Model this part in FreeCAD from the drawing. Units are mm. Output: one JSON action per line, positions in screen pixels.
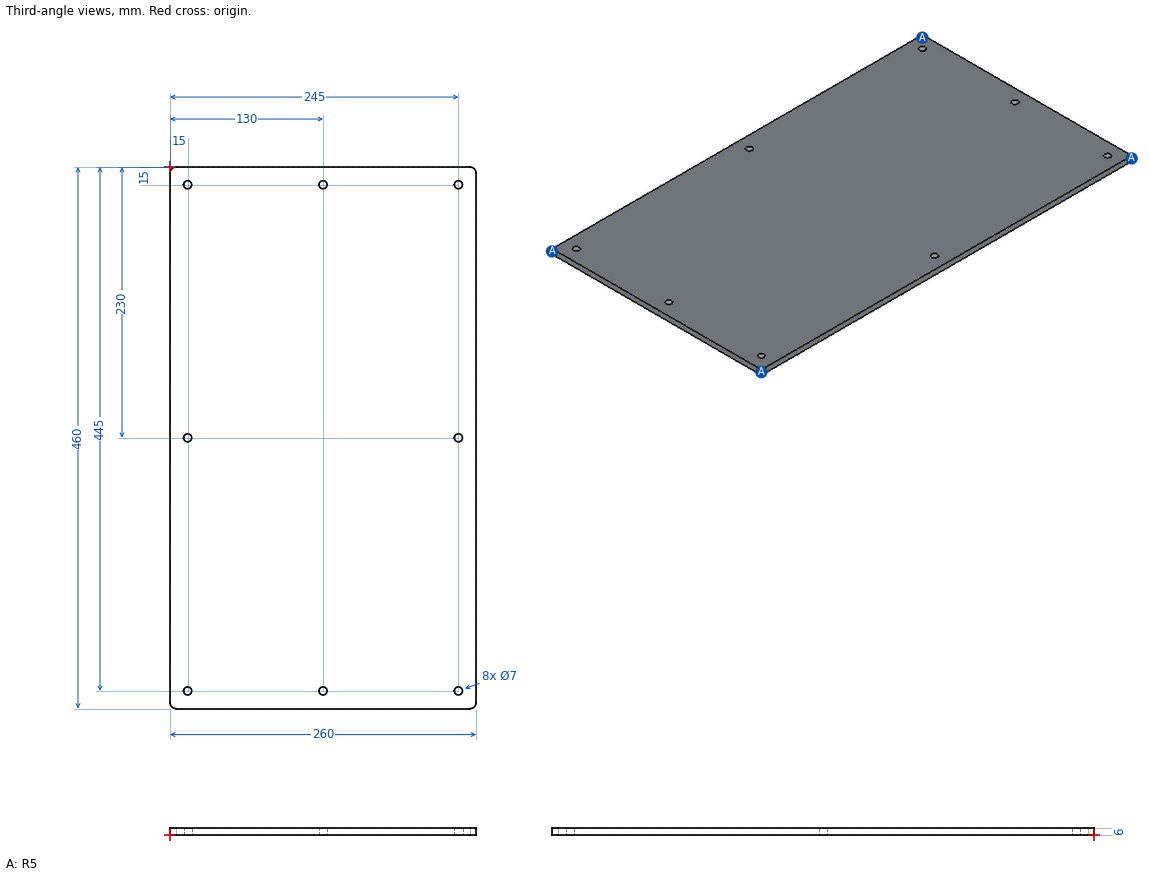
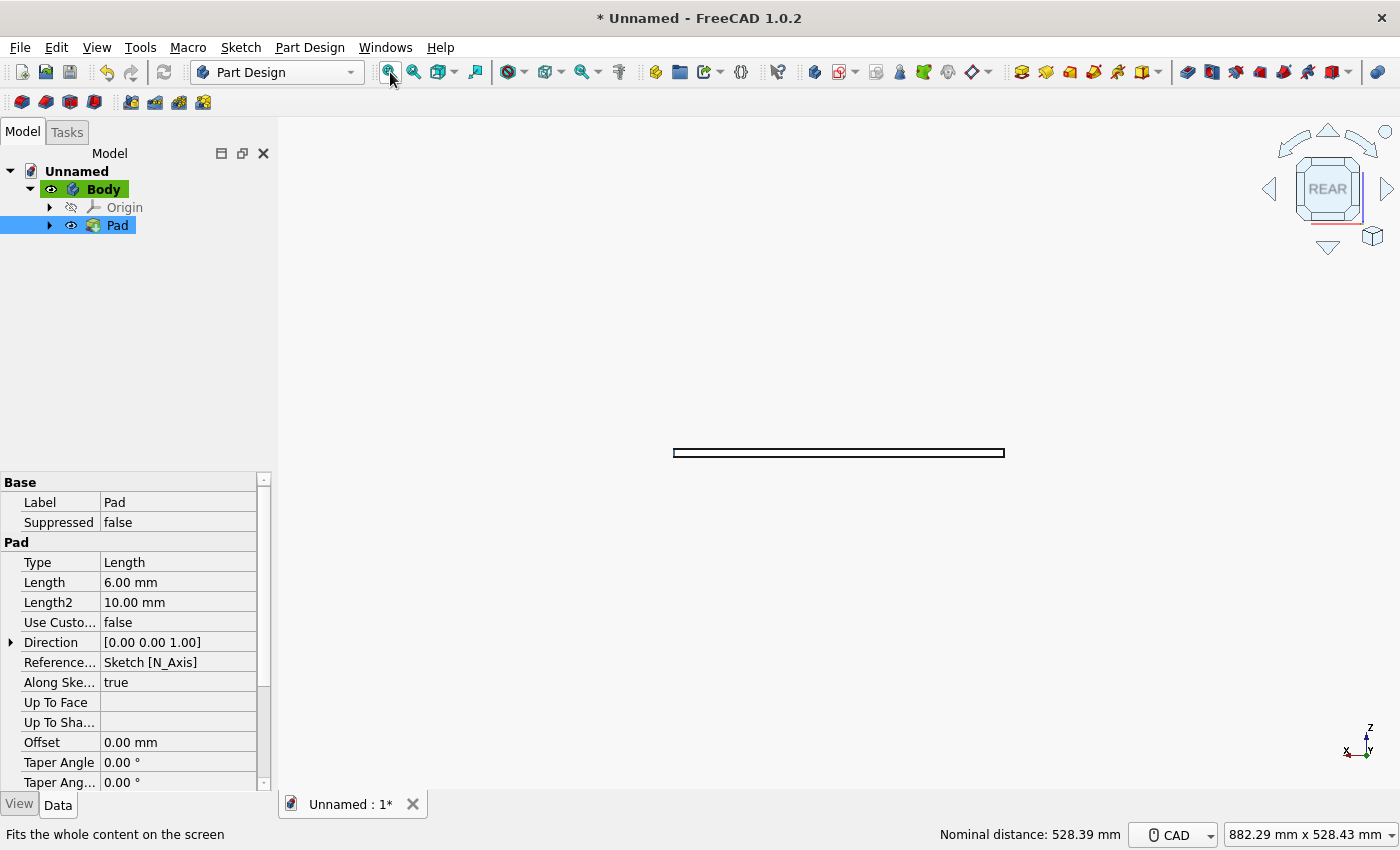
{"action": "scroll", "coordinate": [1004, 452], "scroll_direction": "up", "scroll_amount": 9}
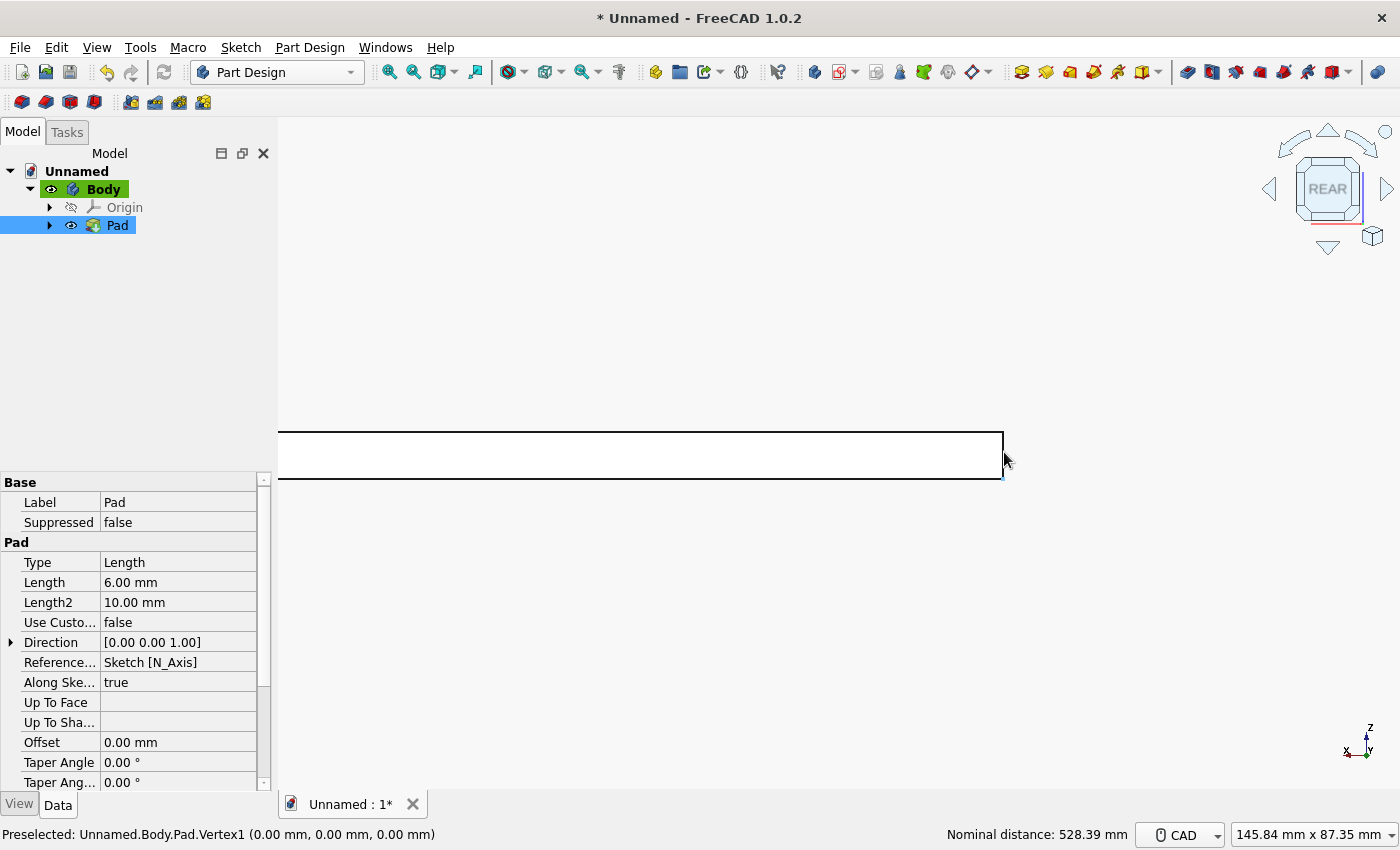
{"action": "left_click", "coordinate": [1003, 455], "text": "ctrl"}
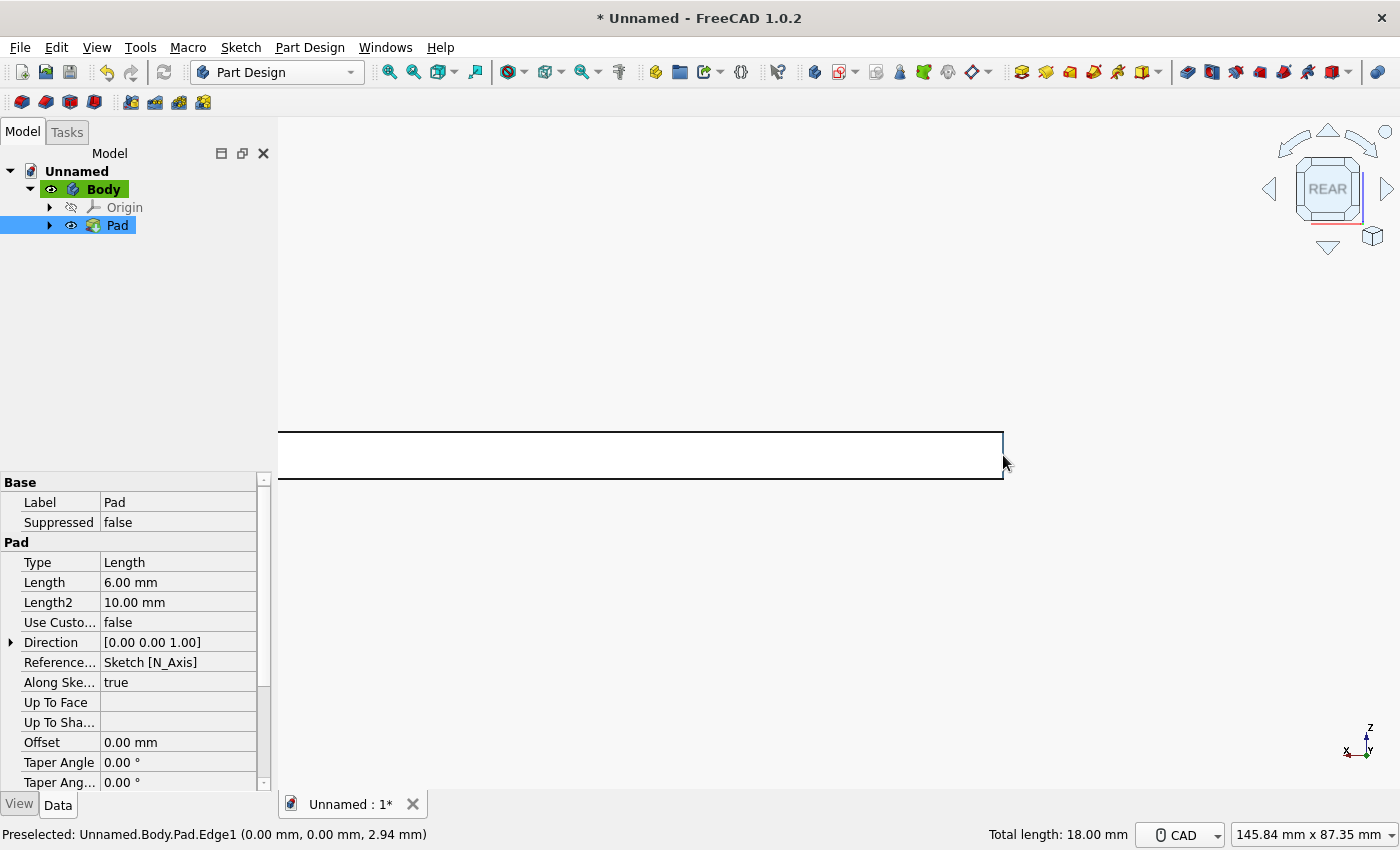
{"action": "left_click", "coordinate": [390, 72]}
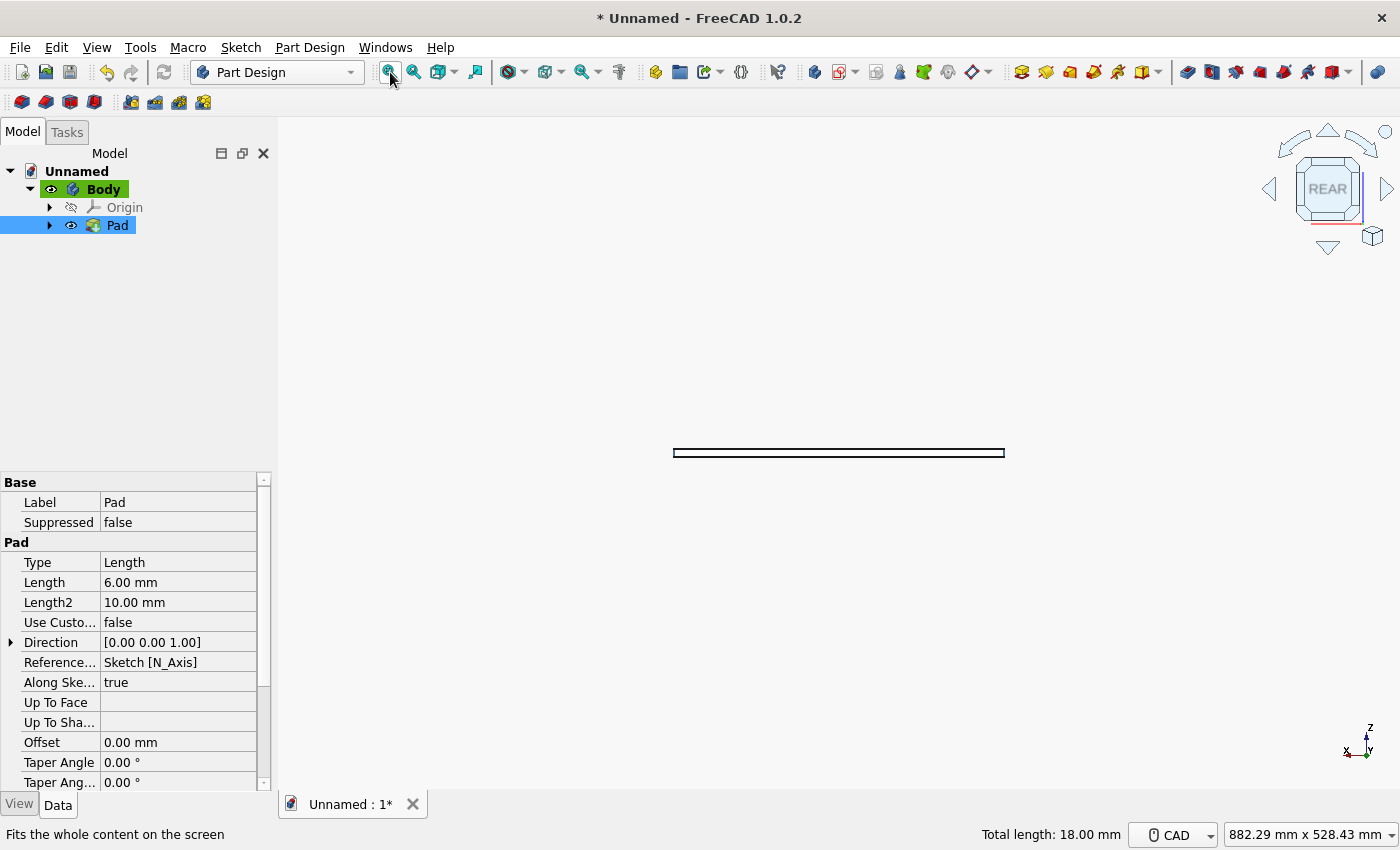
{"action": "key", "text": "6"}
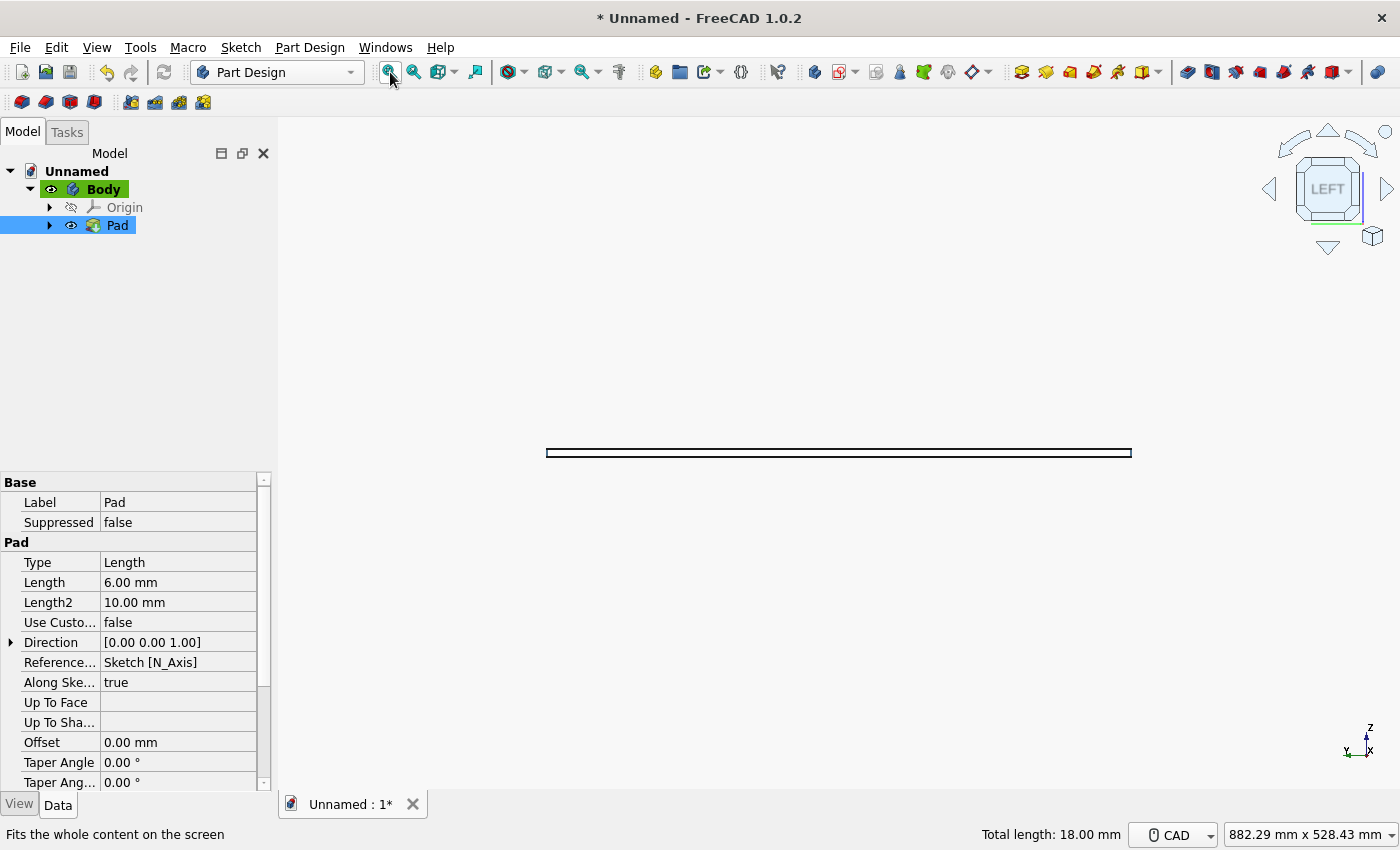
{"action": "scroll", "coordinate": [1131, 452], "scroll_direction": "up", "scroll_amount": 9}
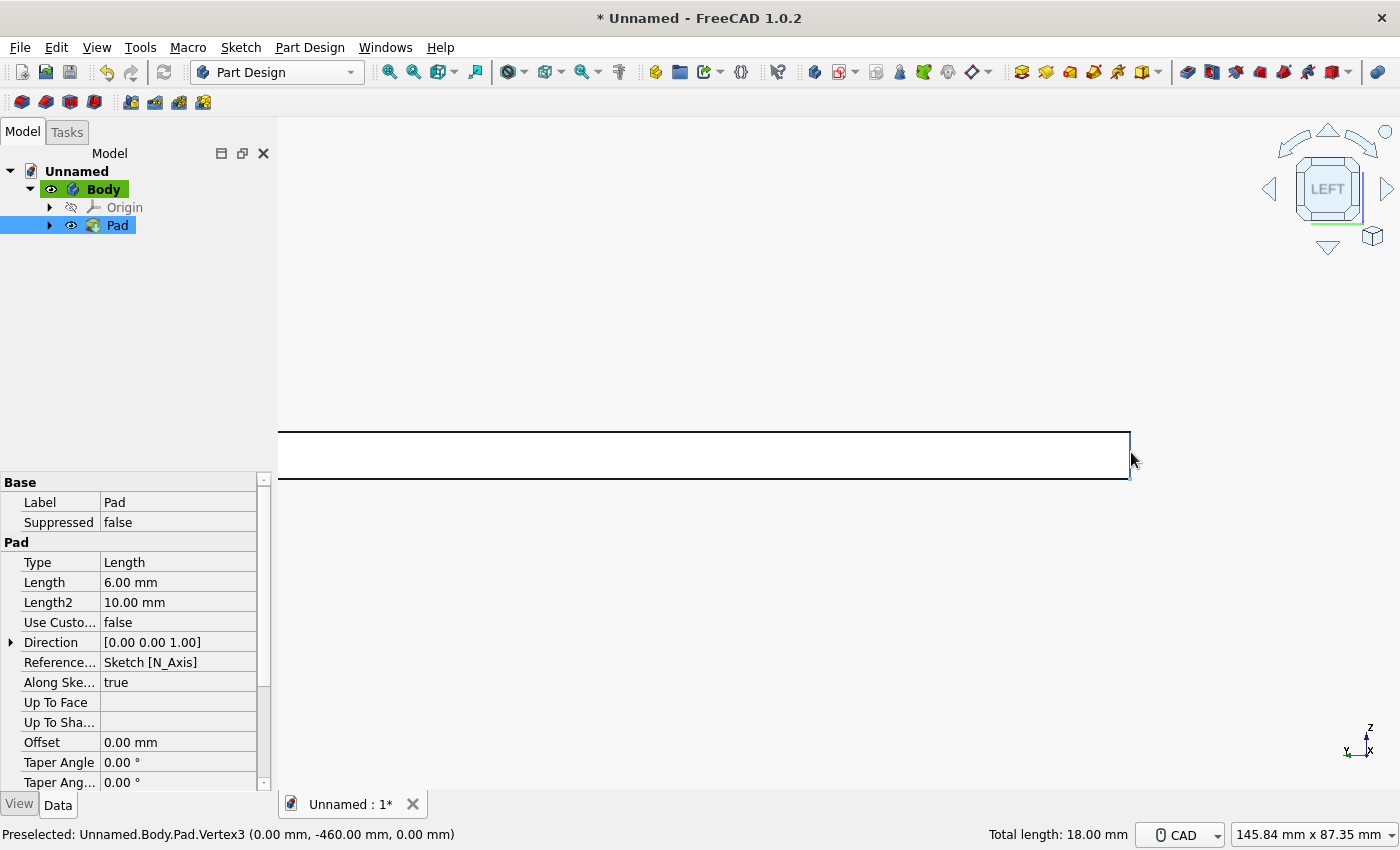
{"action": "key", "text": "v f"}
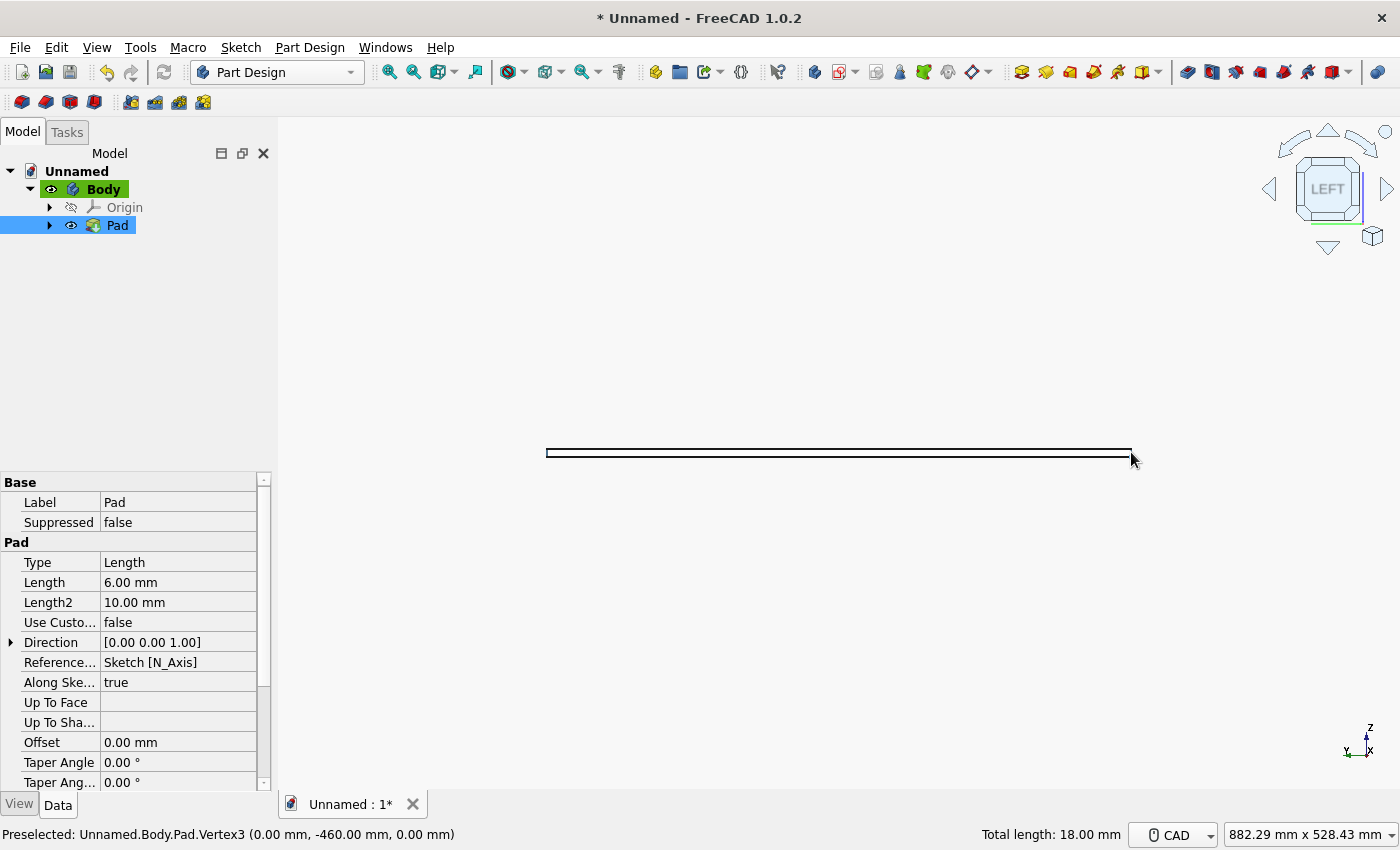
{"action": "key", "text": "v 3"}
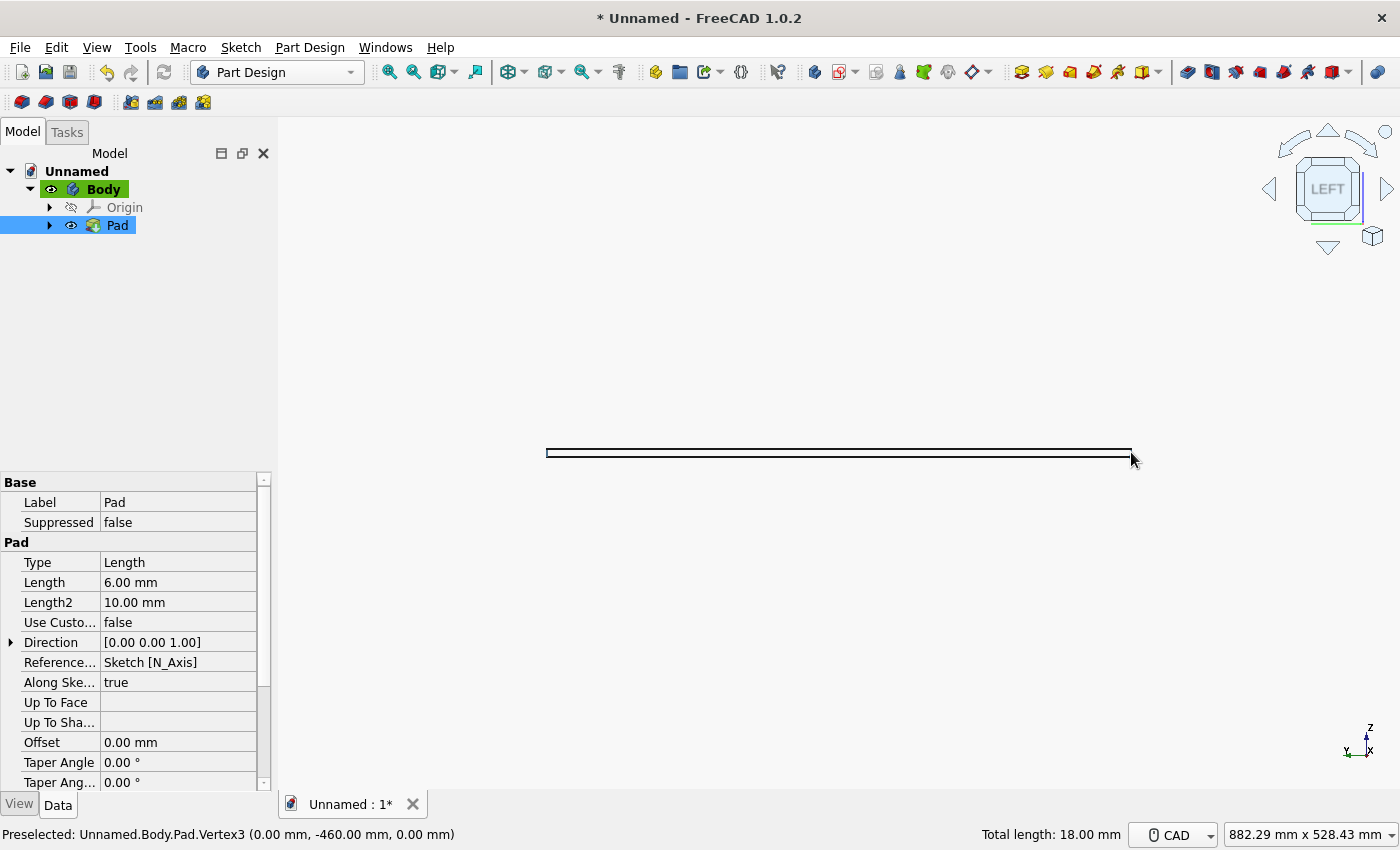
{"action": "key", "text": "0"}